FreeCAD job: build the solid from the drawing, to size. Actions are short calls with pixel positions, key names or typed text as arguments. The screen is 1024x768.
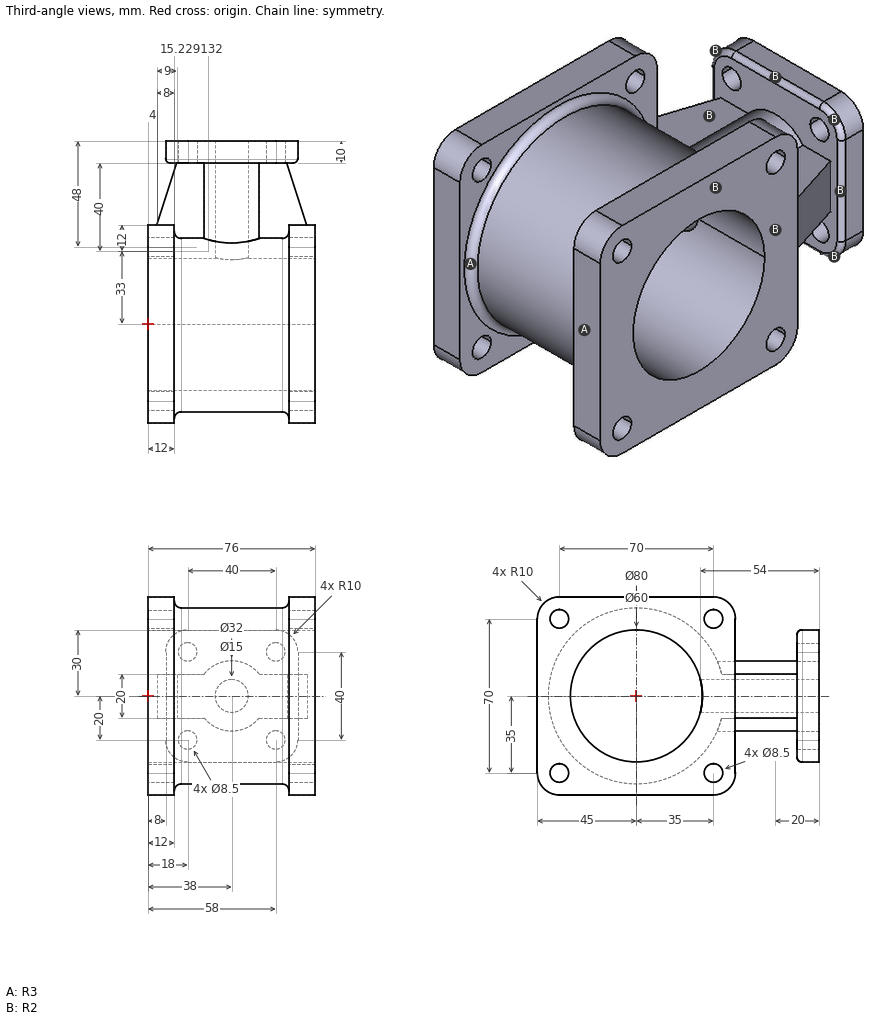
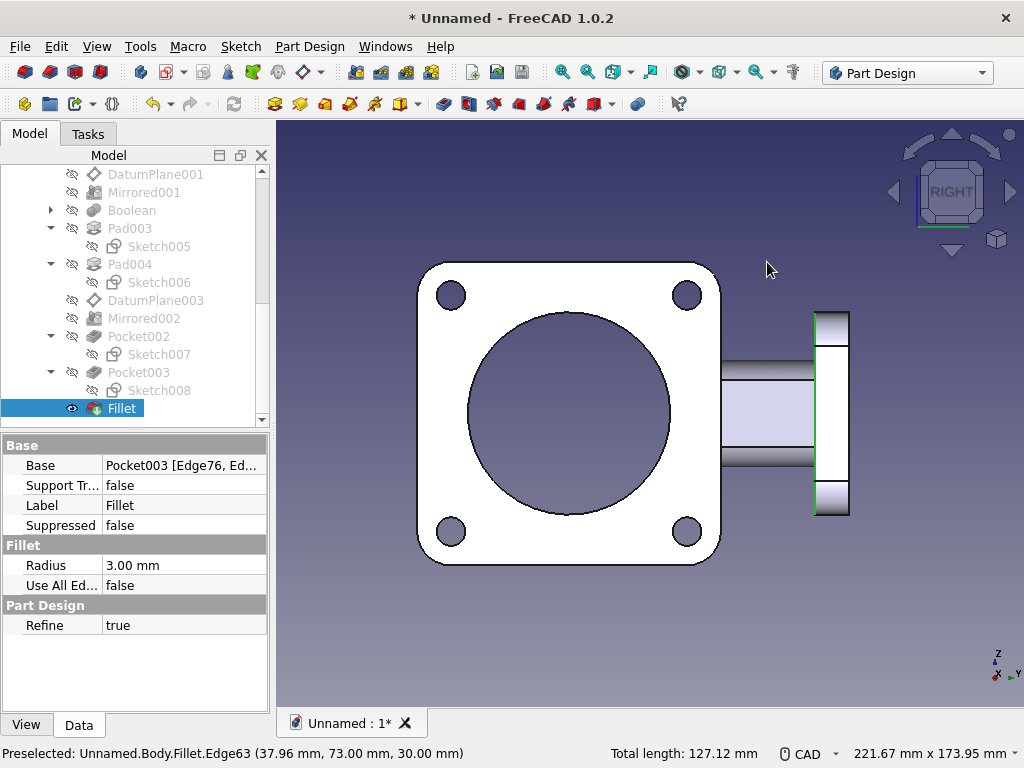
key(5)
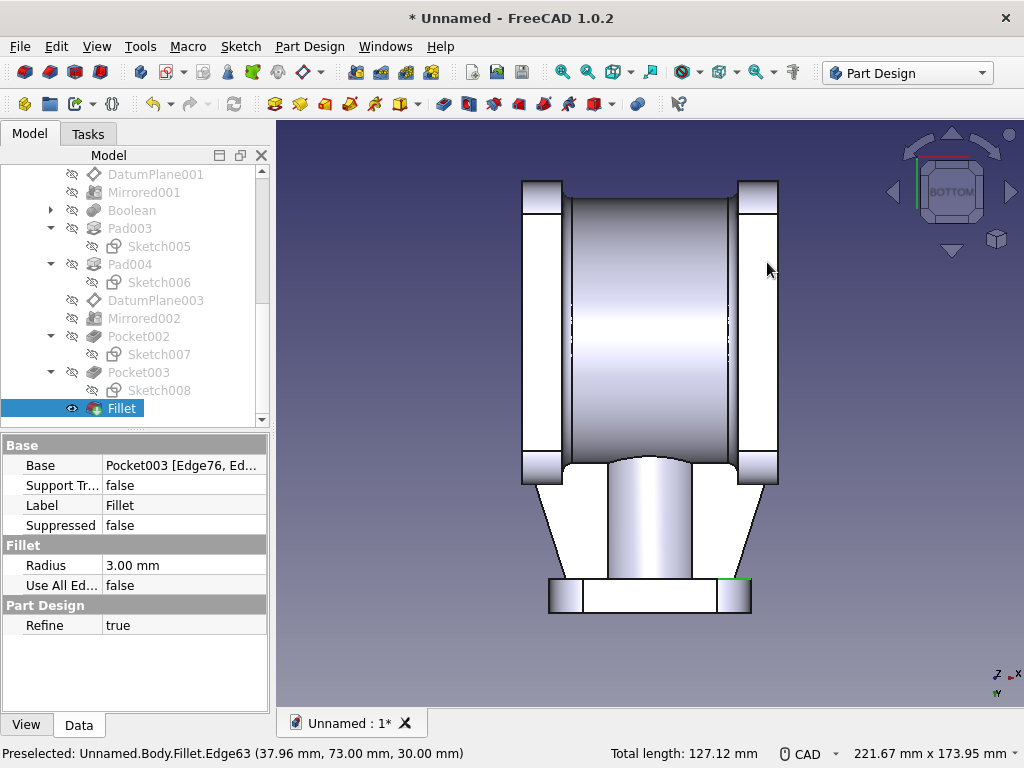
click(559, 578, ctrl)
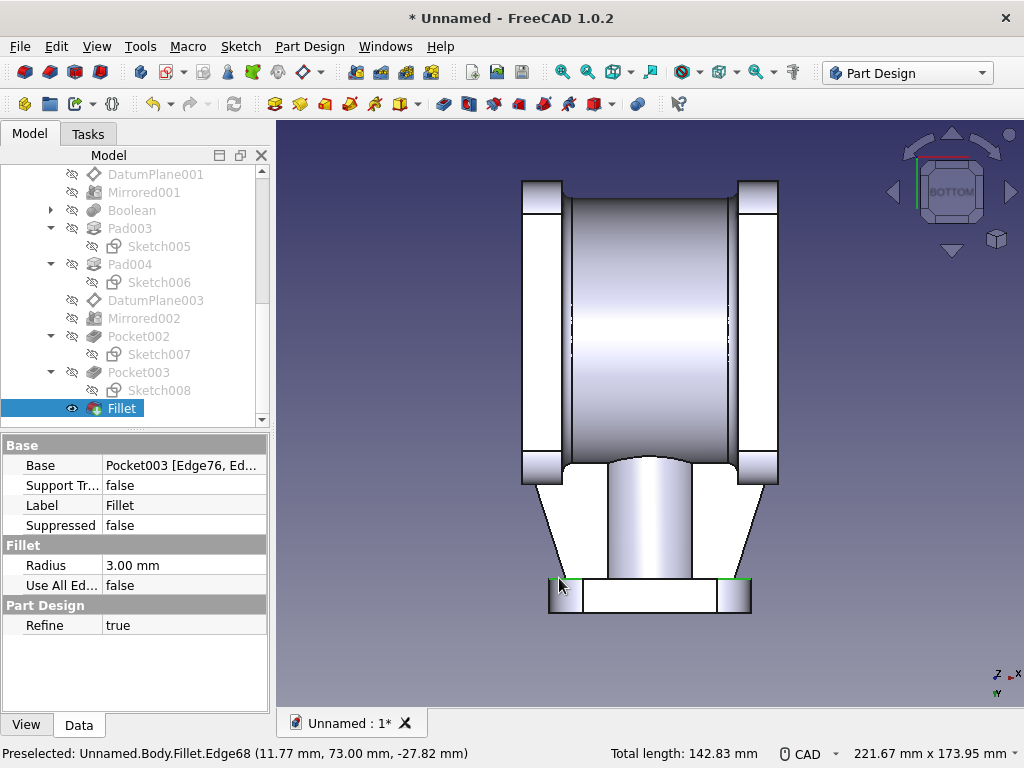
click(650, 578, ctrl)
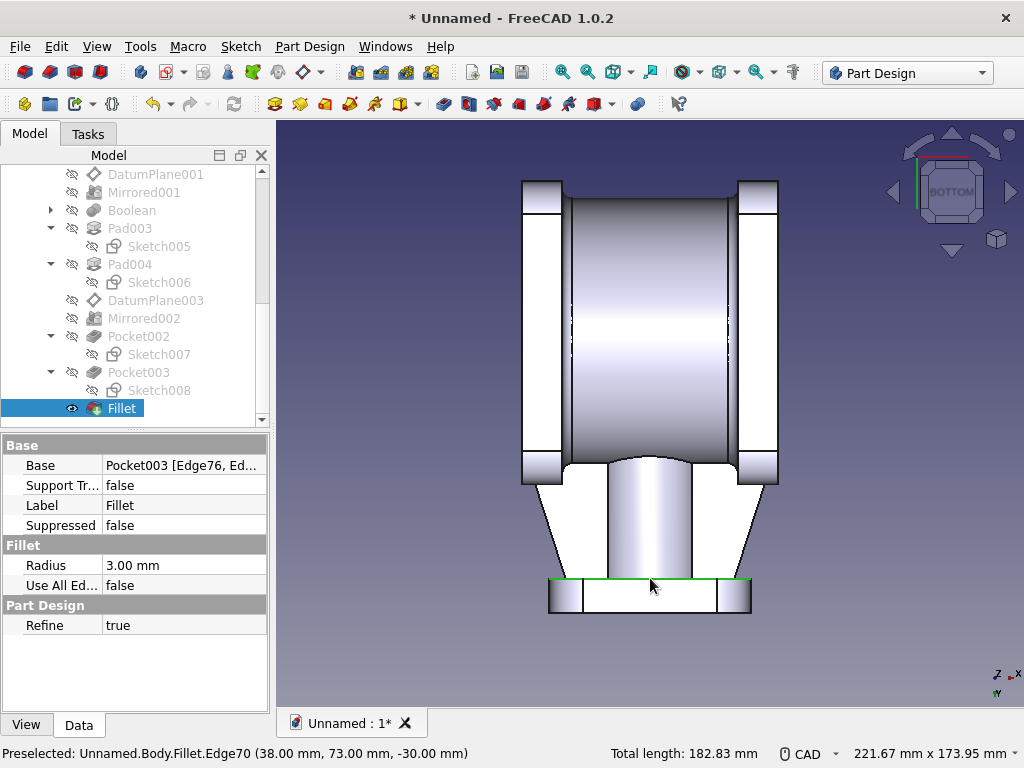
key(4)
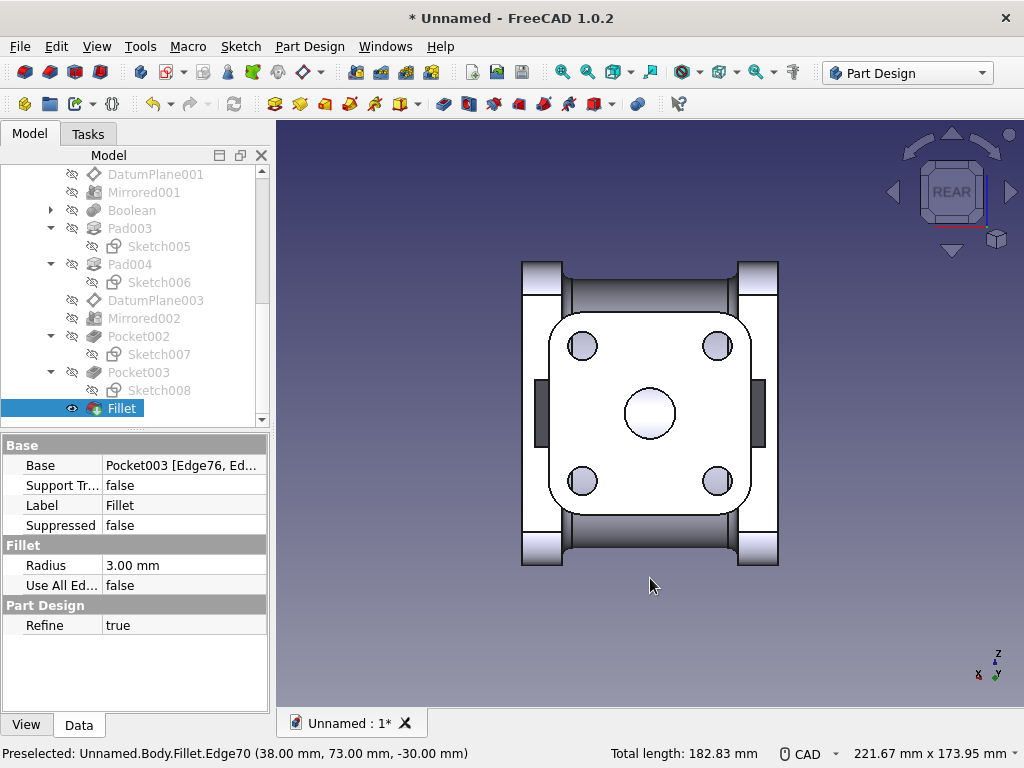
key(6)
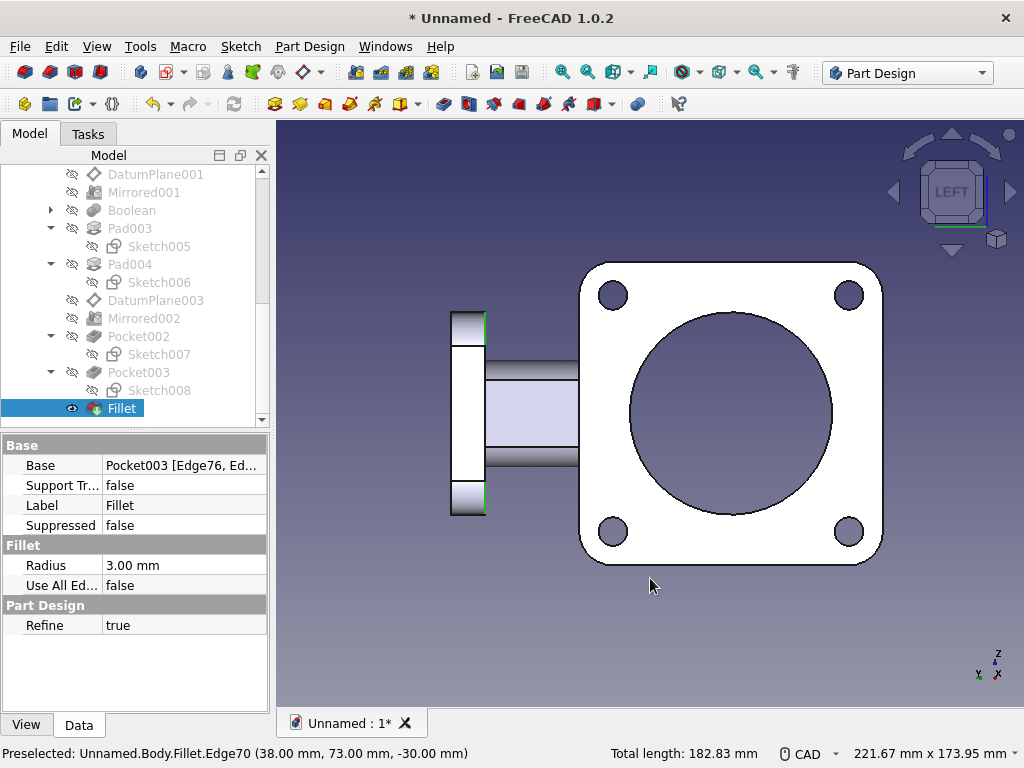
click(485, 413, ctrl)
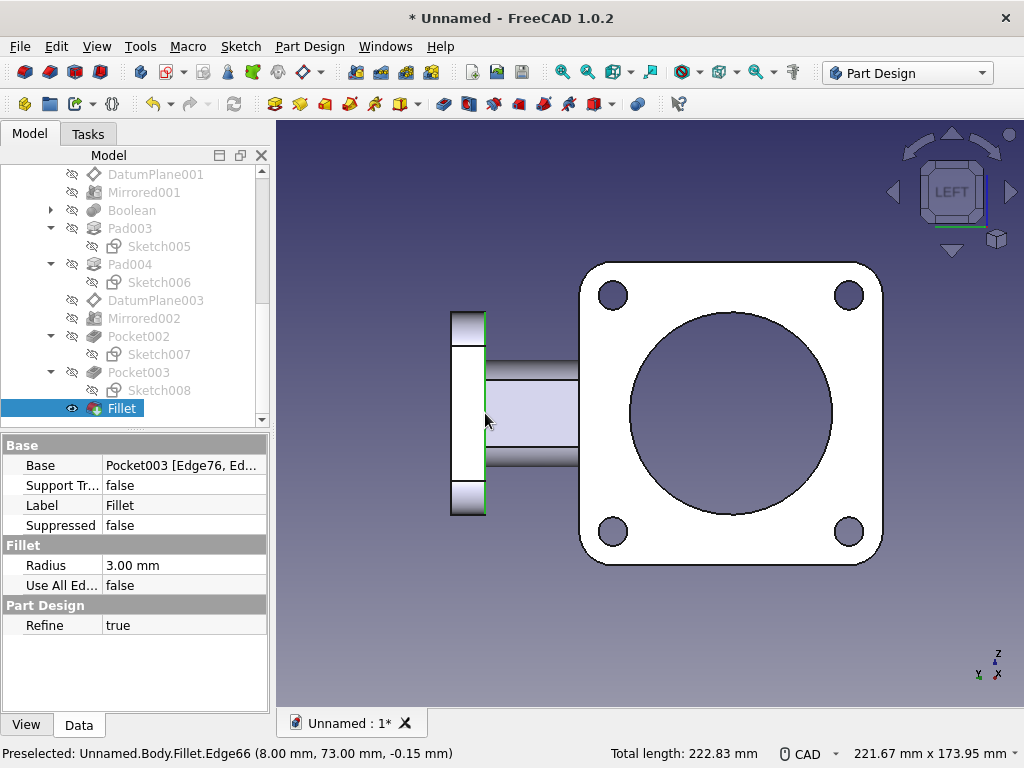
click(25, 72)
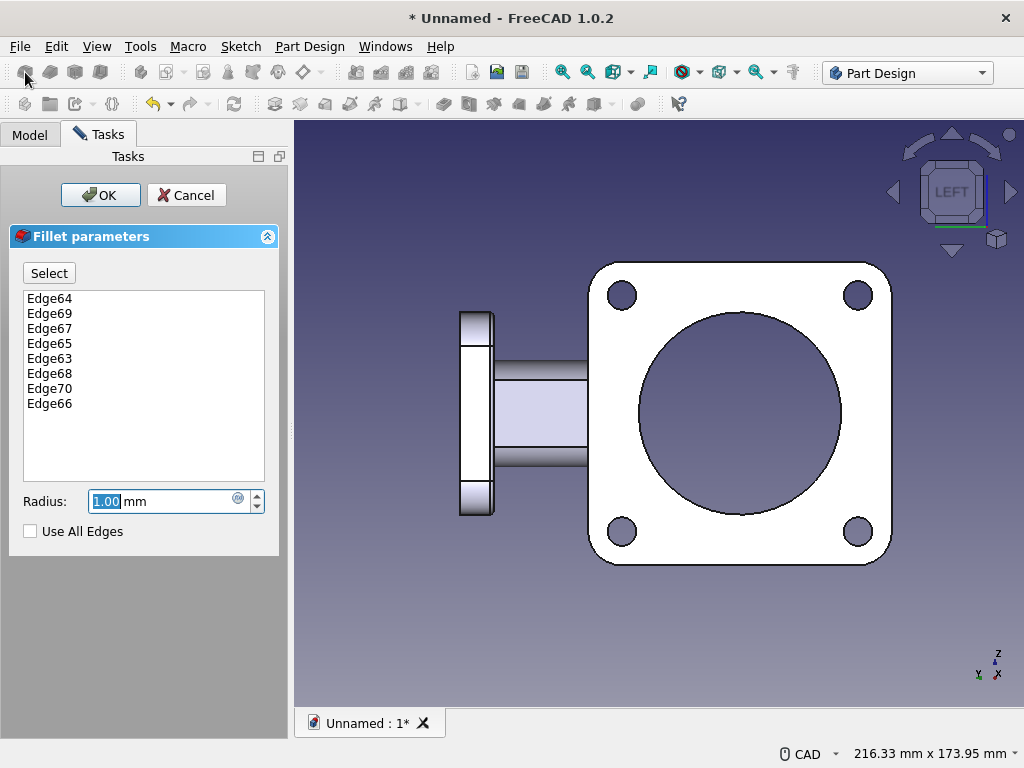
text(2)
key(Tab)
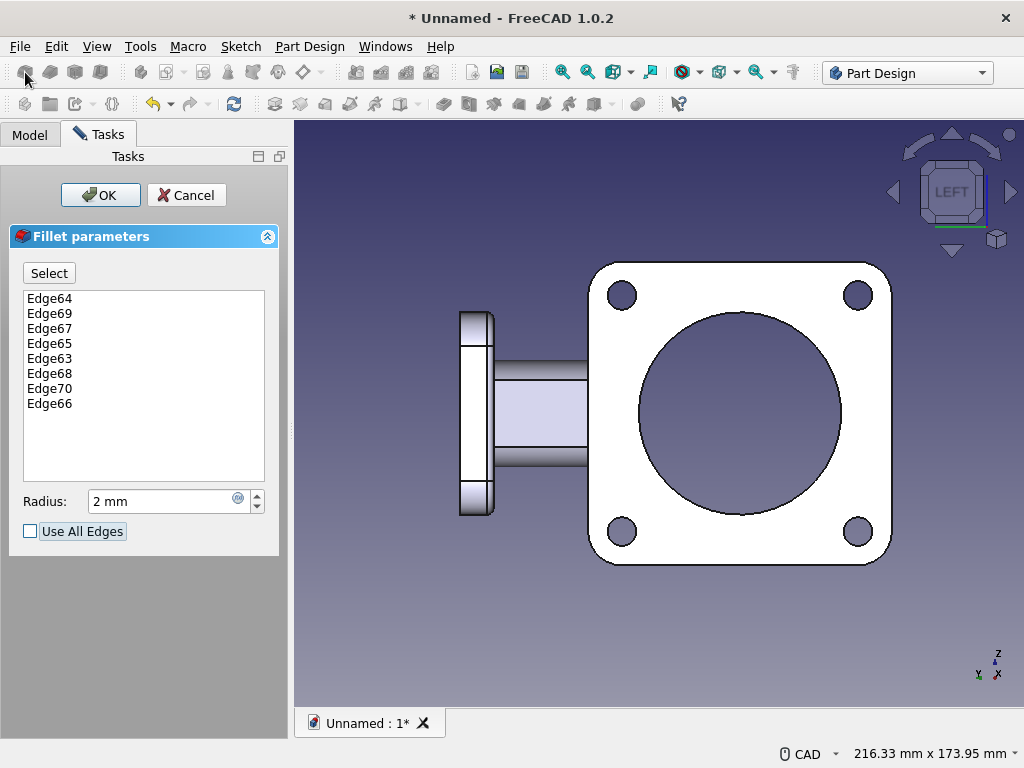
click(101, 195)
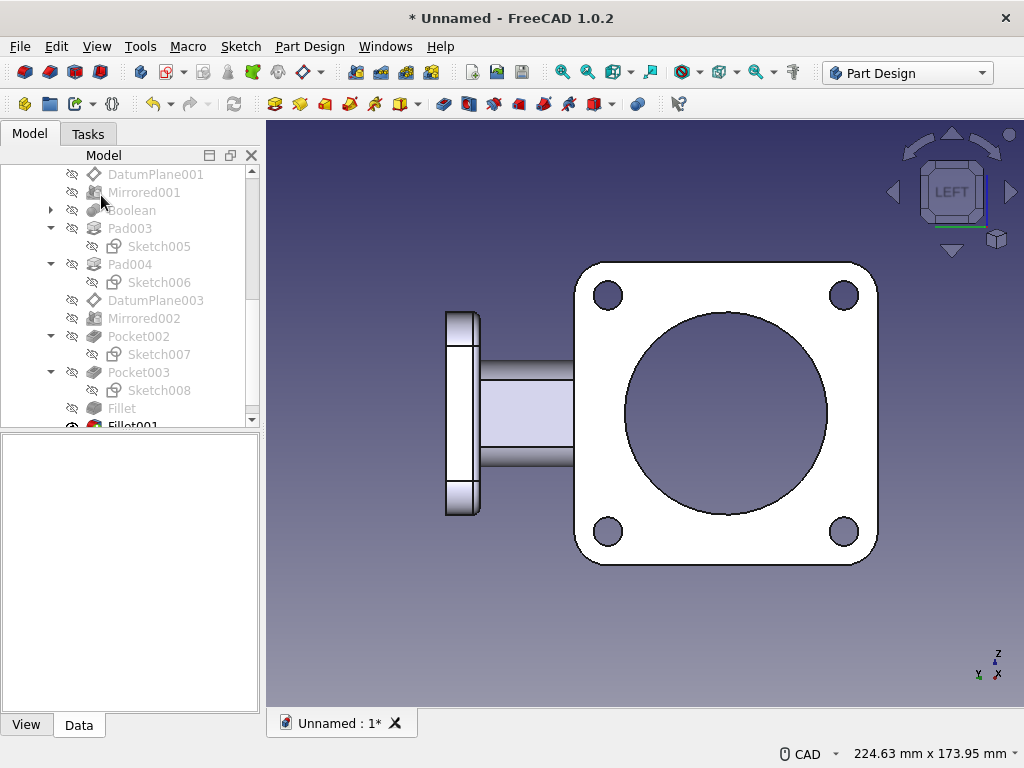
key(0)